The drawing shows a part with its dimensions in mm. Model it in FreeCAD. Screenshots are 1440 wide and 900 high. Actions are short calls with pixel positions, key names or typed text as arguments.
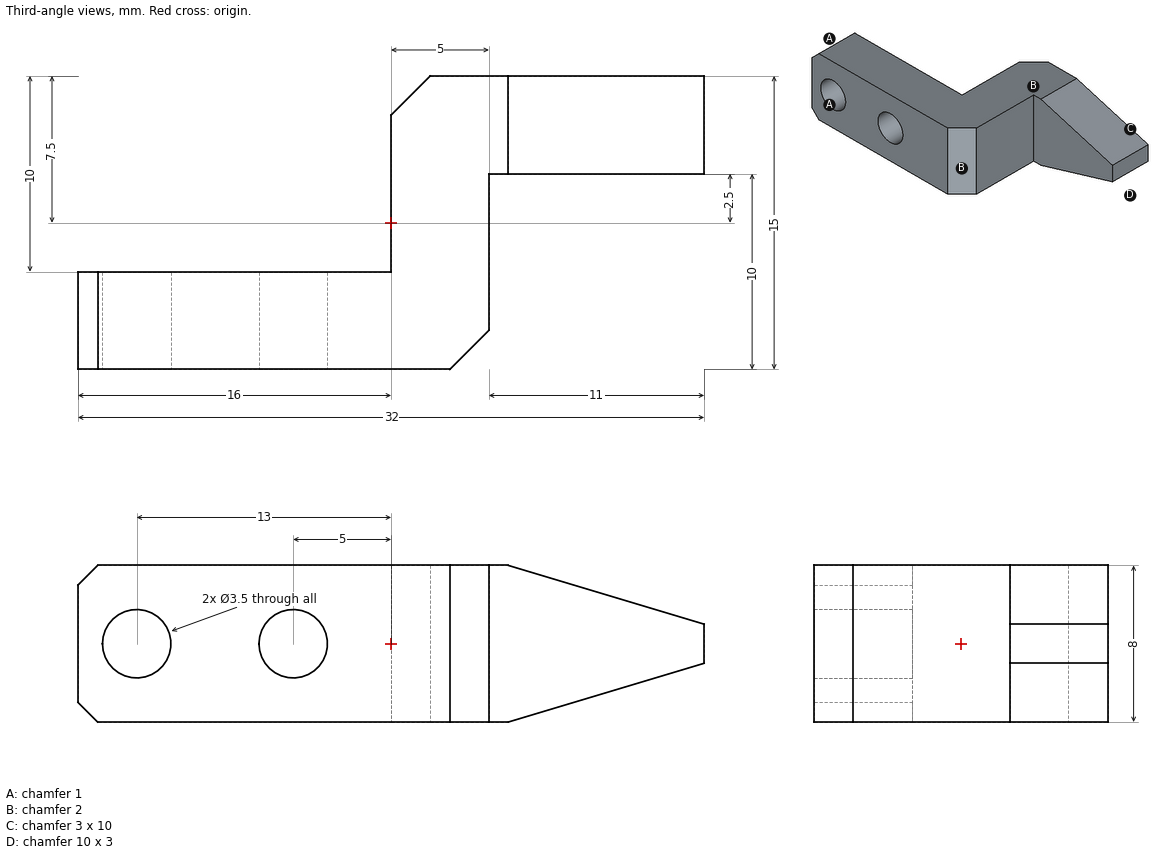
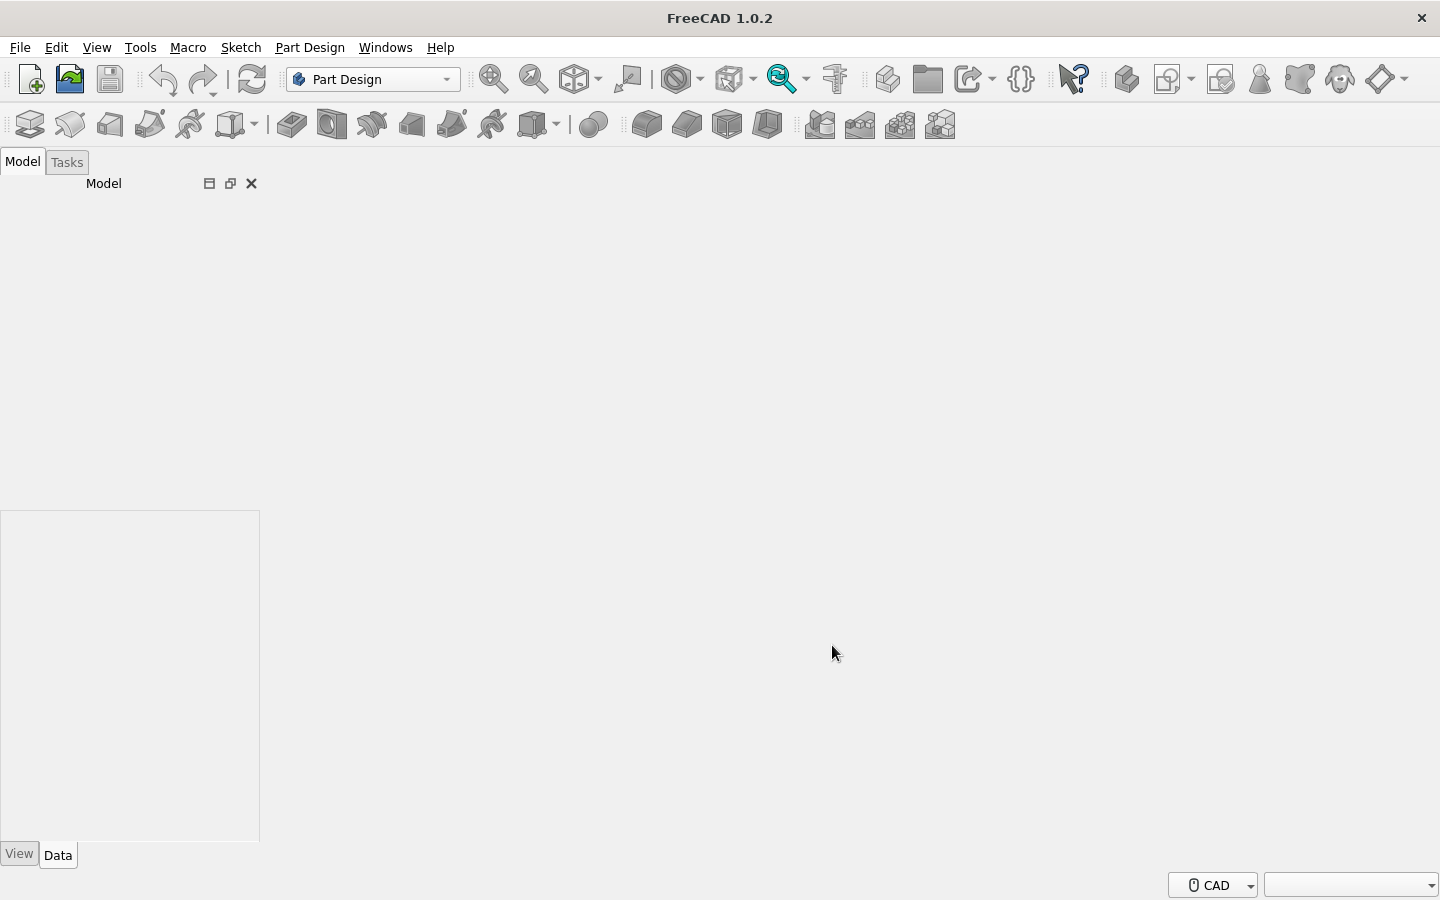
key(ctrl+n)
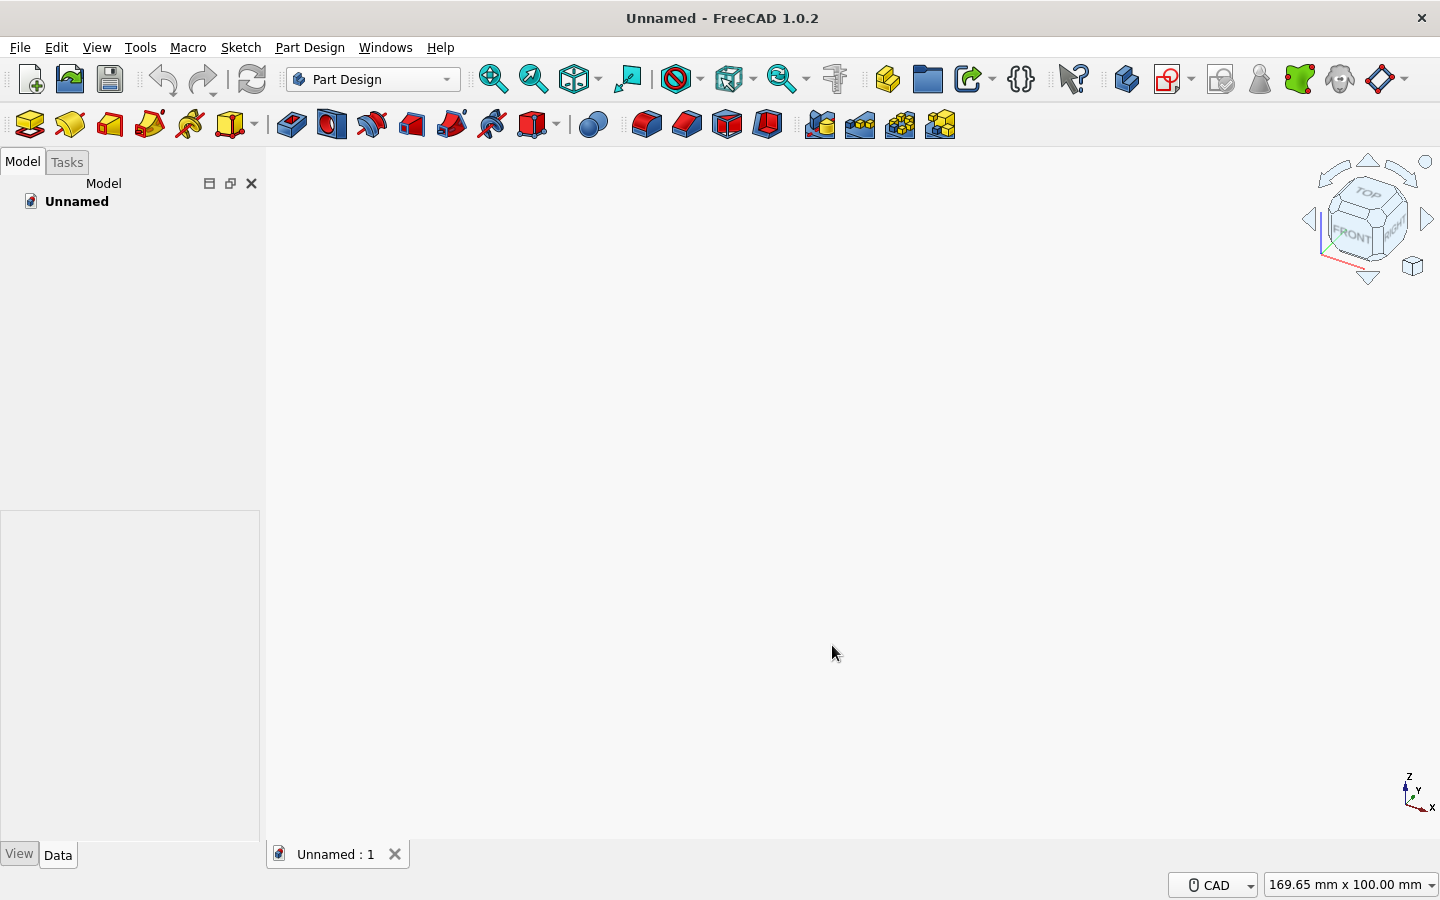
click(1168, 80)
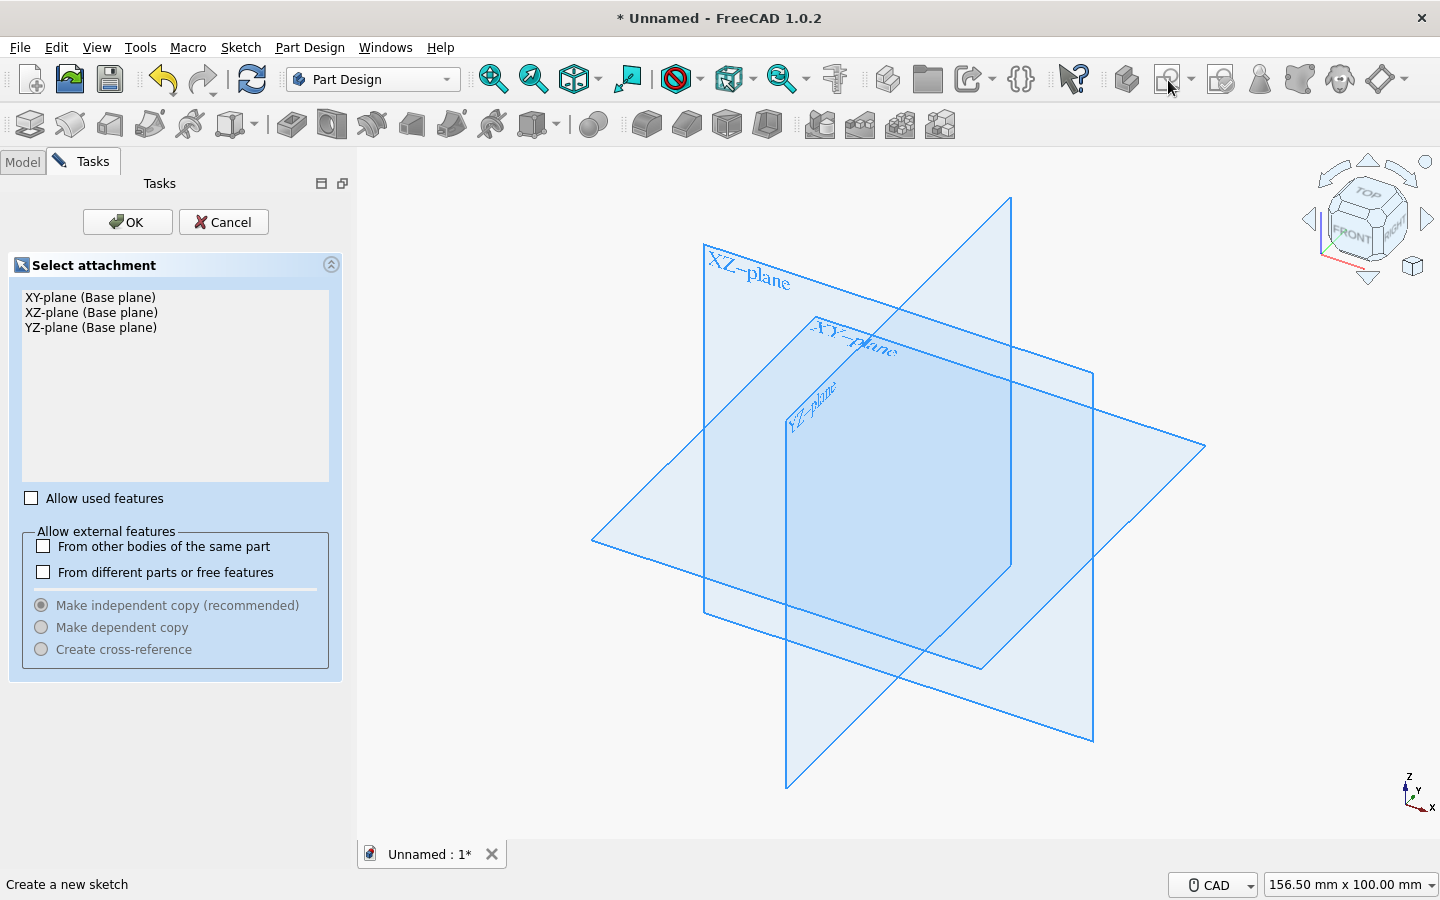
click(82, 298)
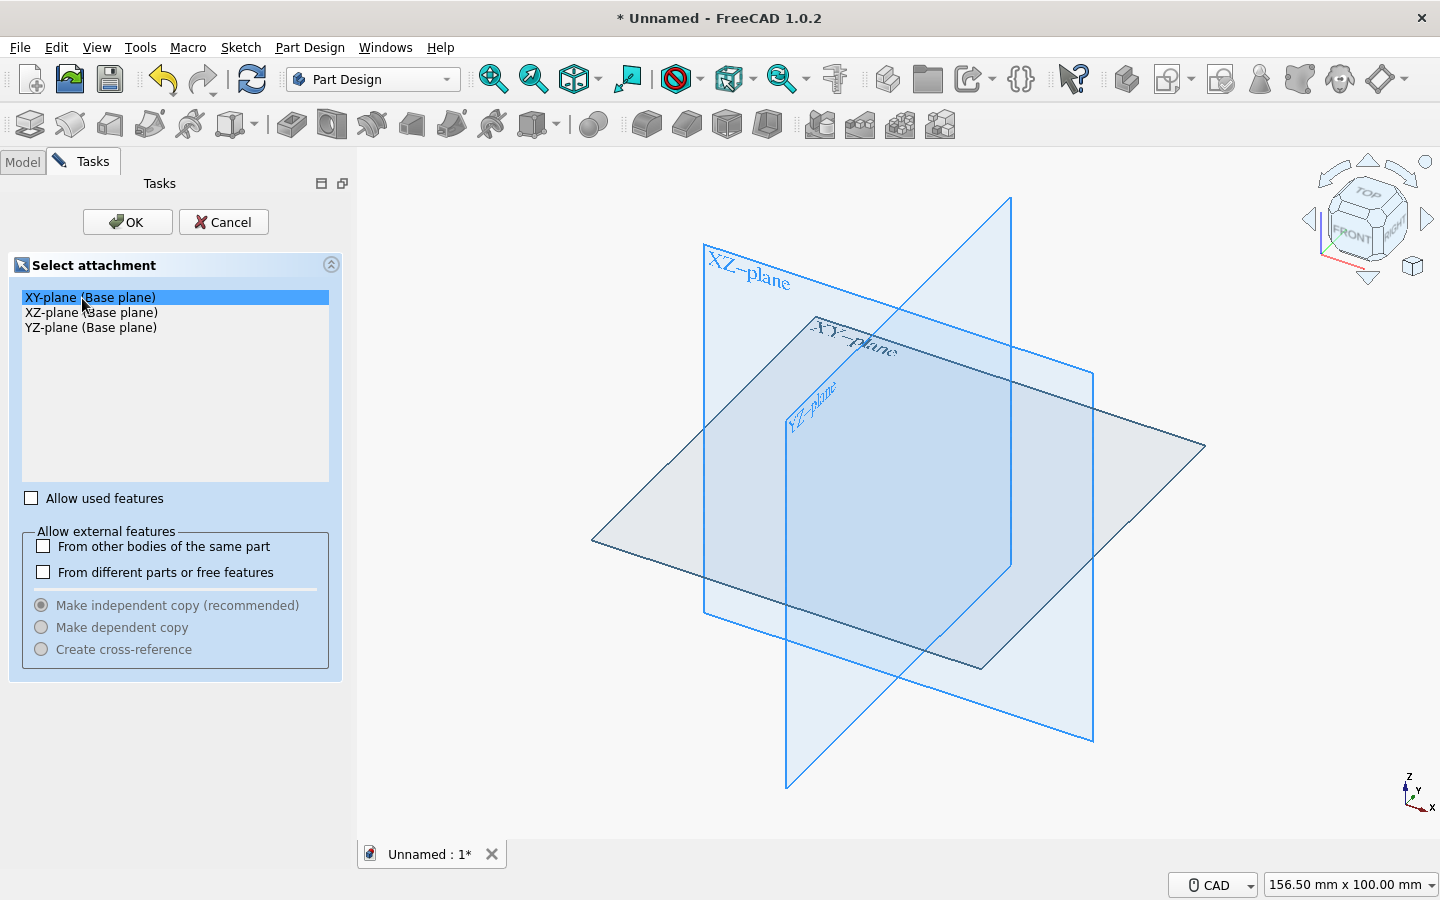
click(128, 222)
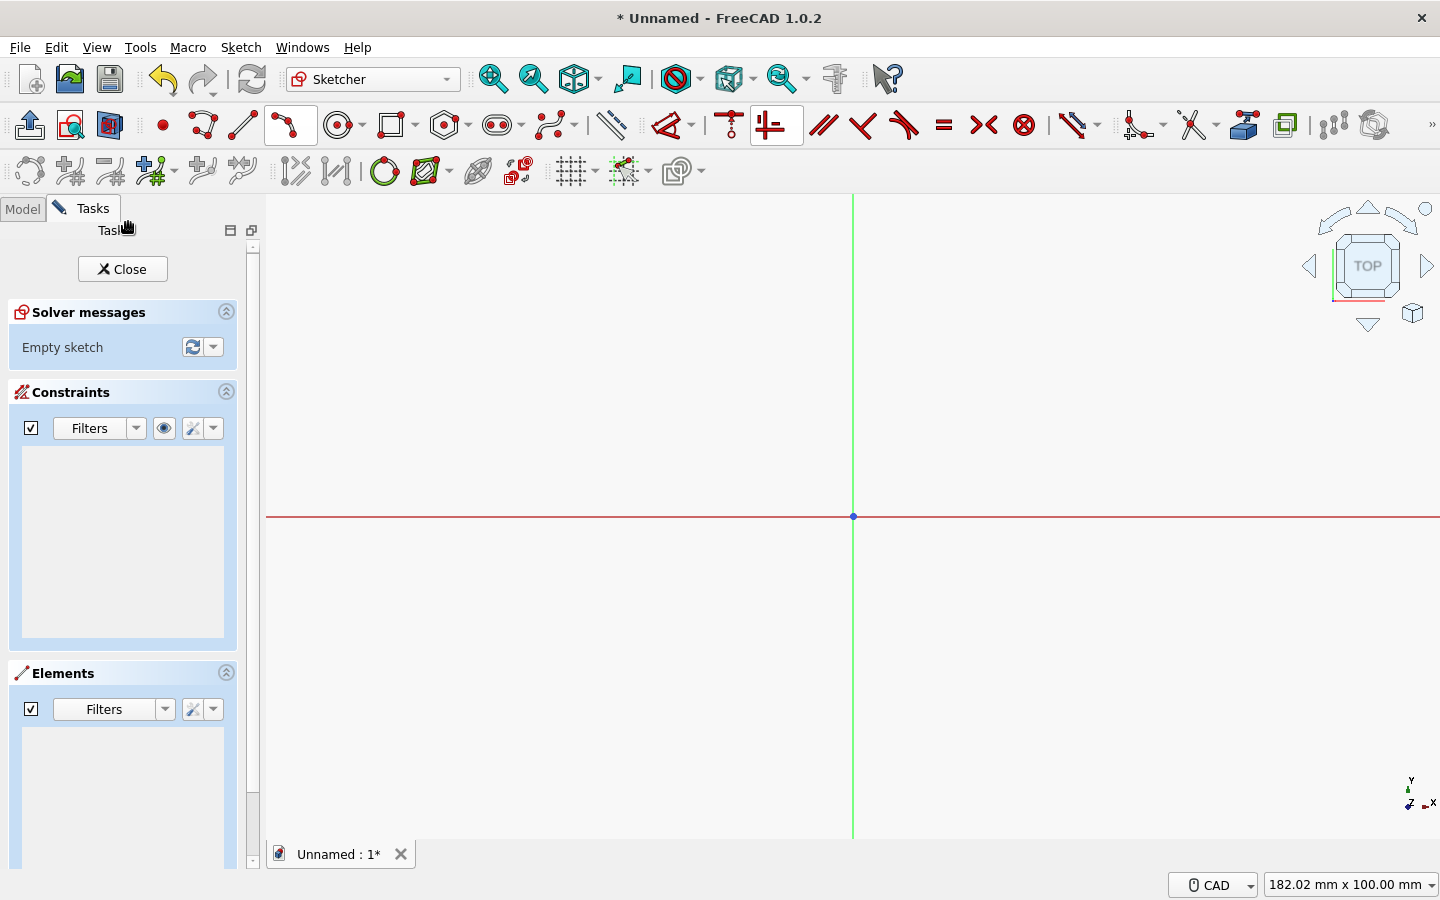
scroll(883, 516, up, 6)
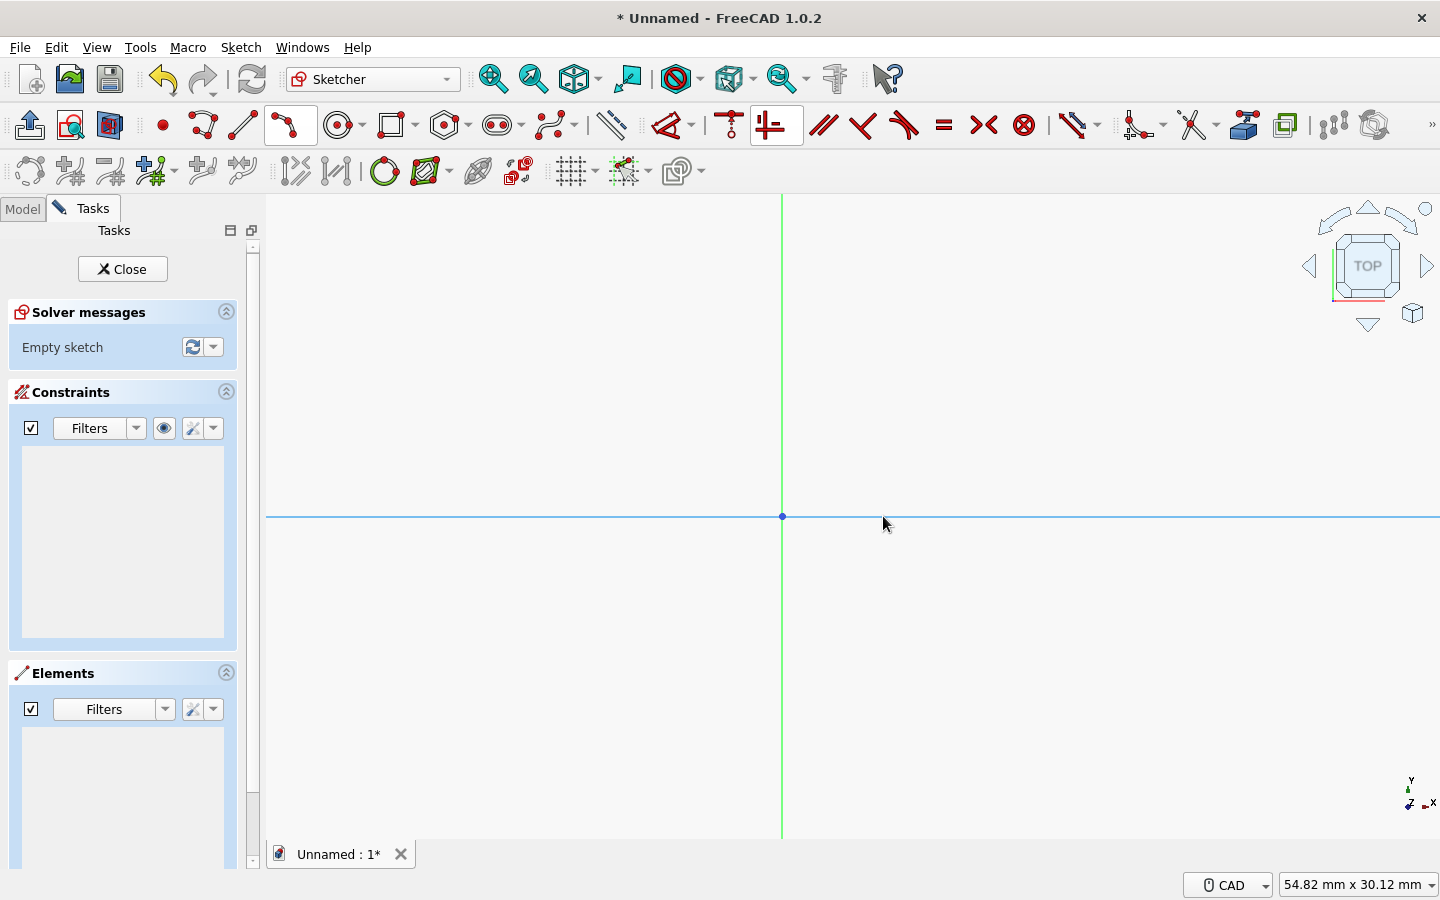
key(g)
key(v)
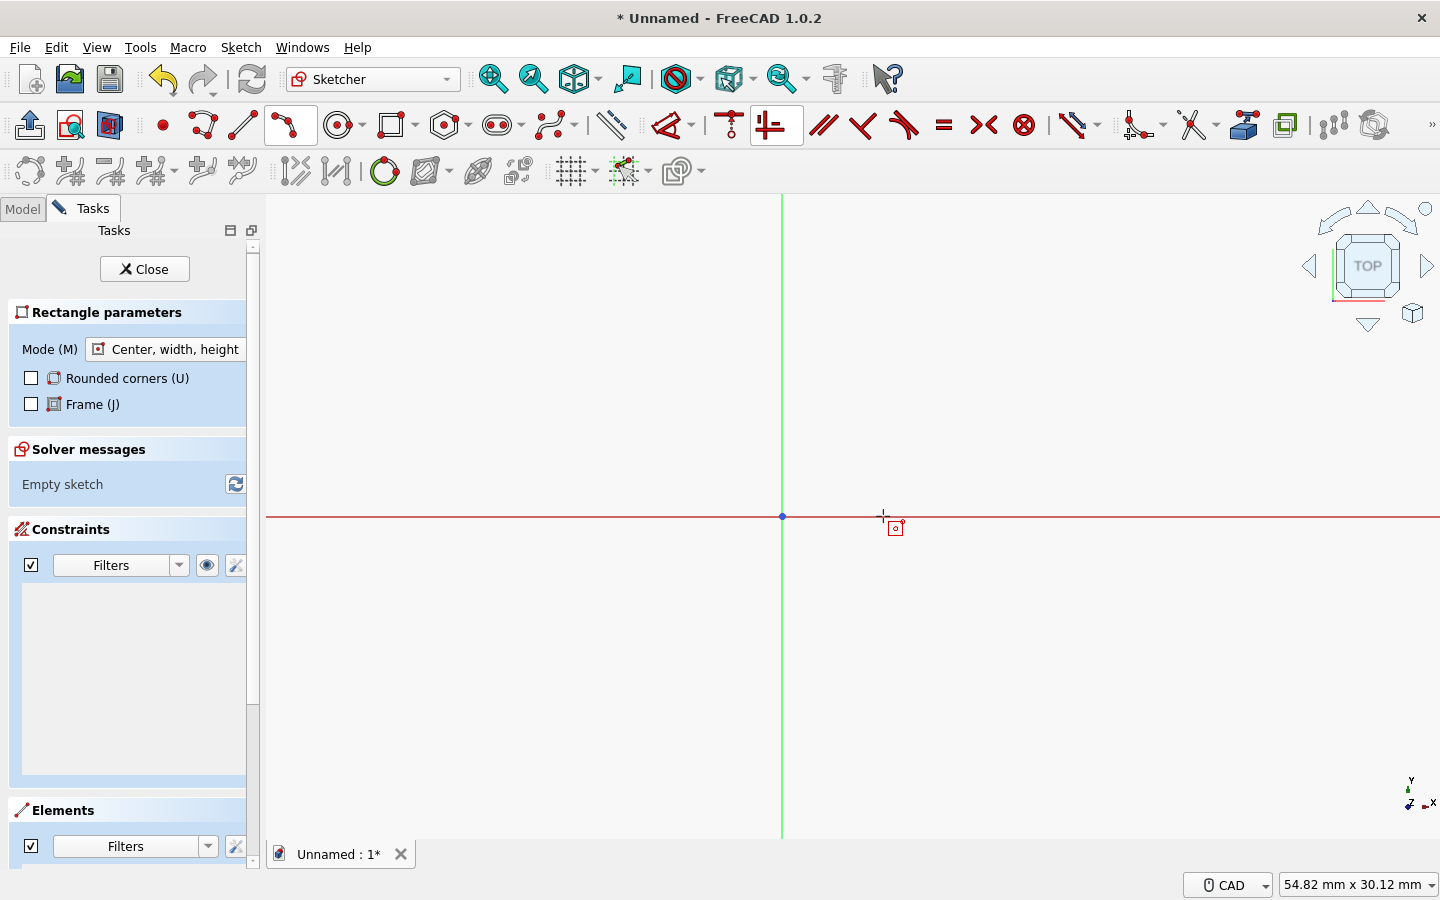
click(782, 516)
move(1125, 356)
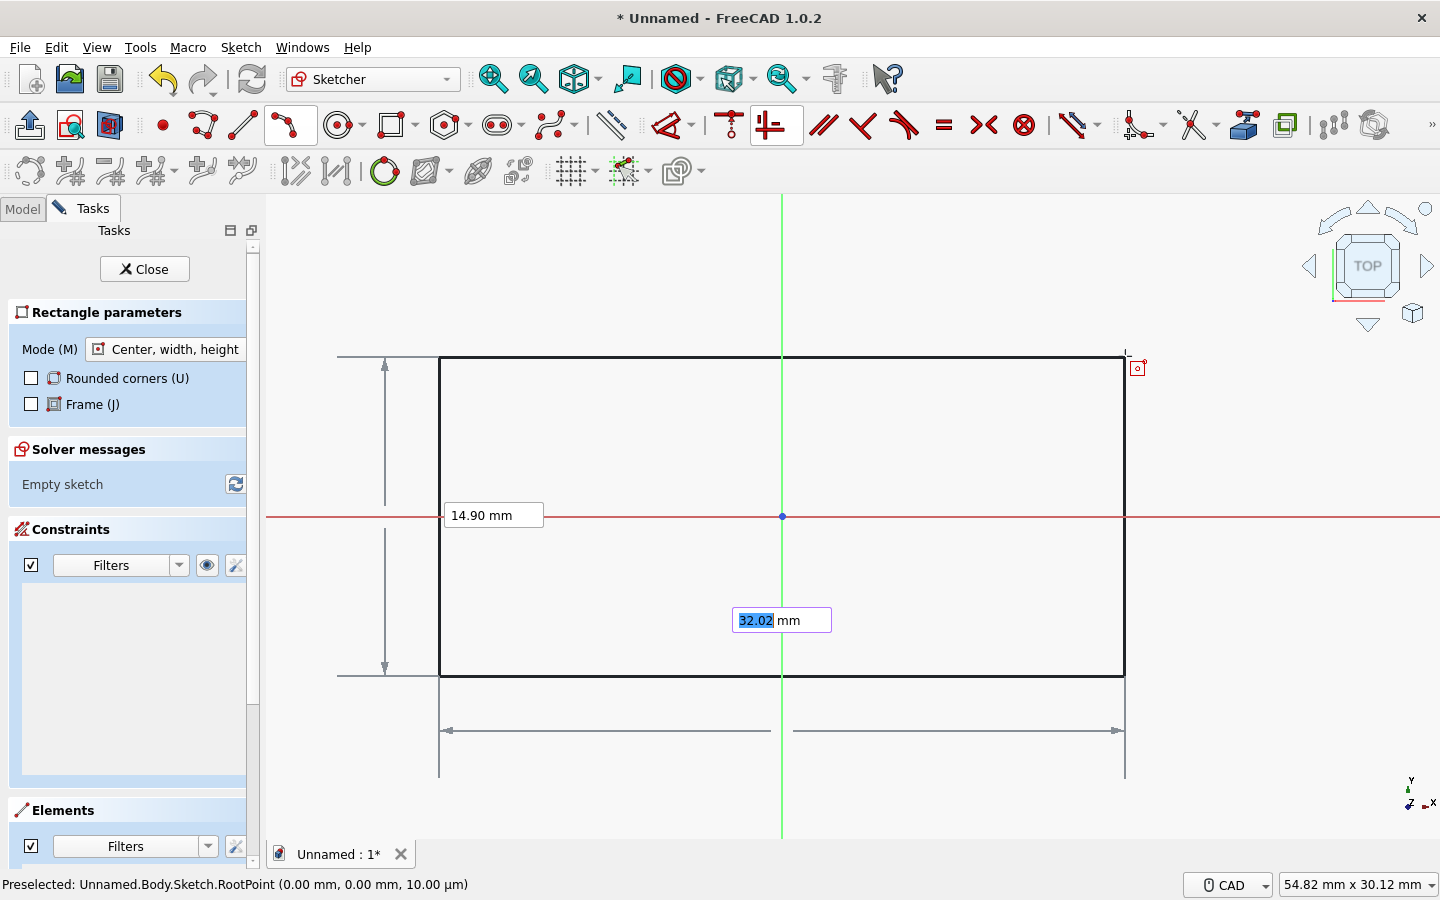
text(32)
key(Tab)
text(15)
key(Return)
key(Escape)